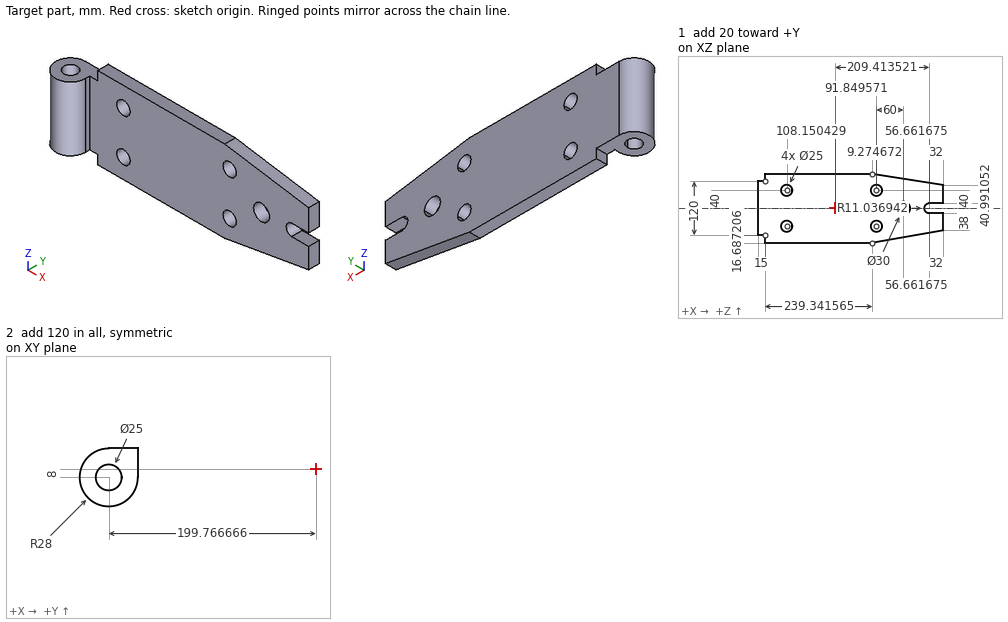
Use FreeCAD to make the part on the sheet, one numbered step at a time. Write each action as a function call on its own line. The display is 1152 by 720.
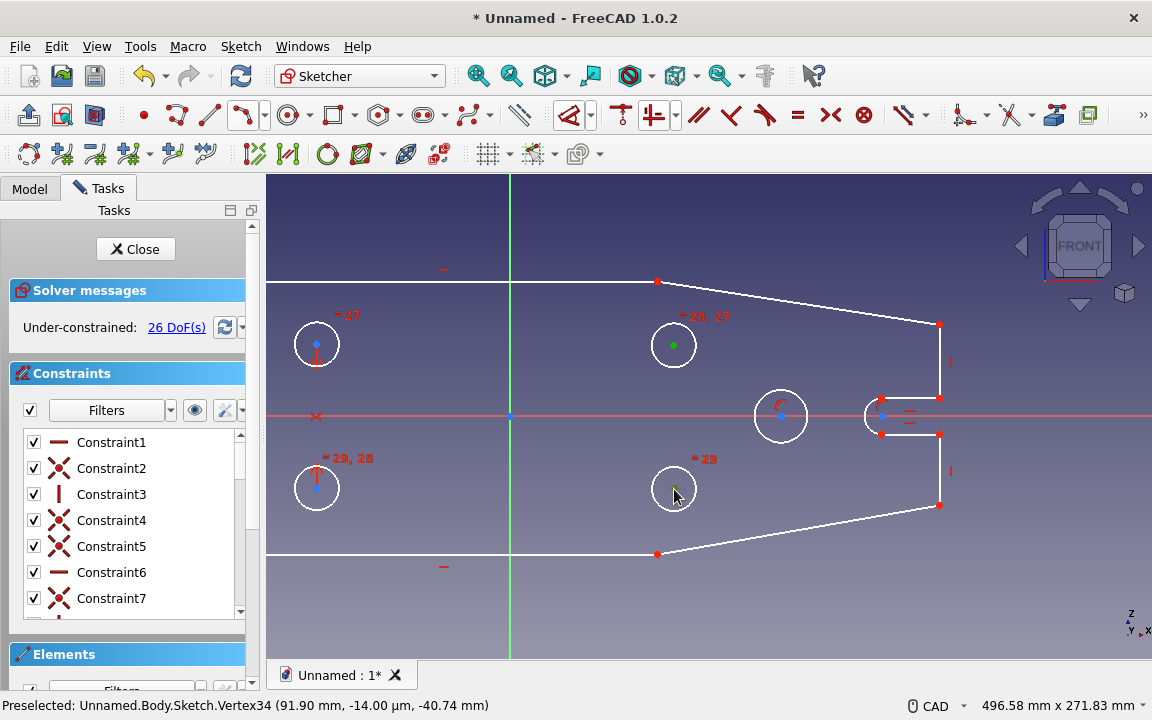
click(344, 416)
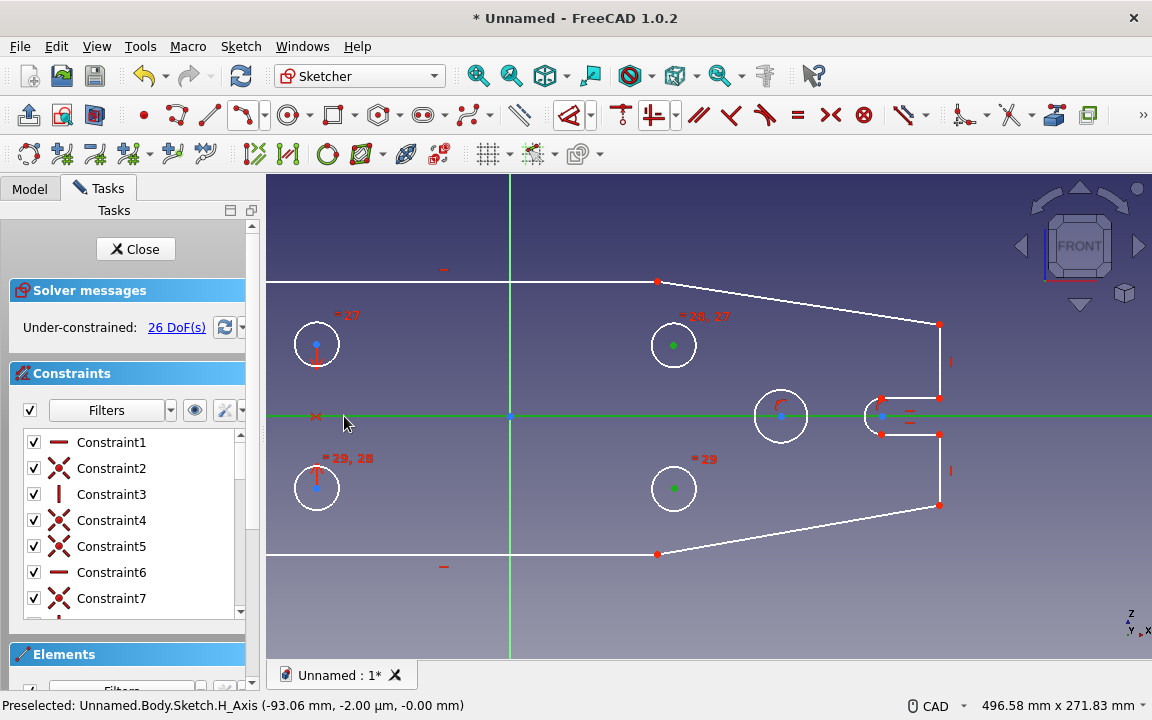
click(831, 116)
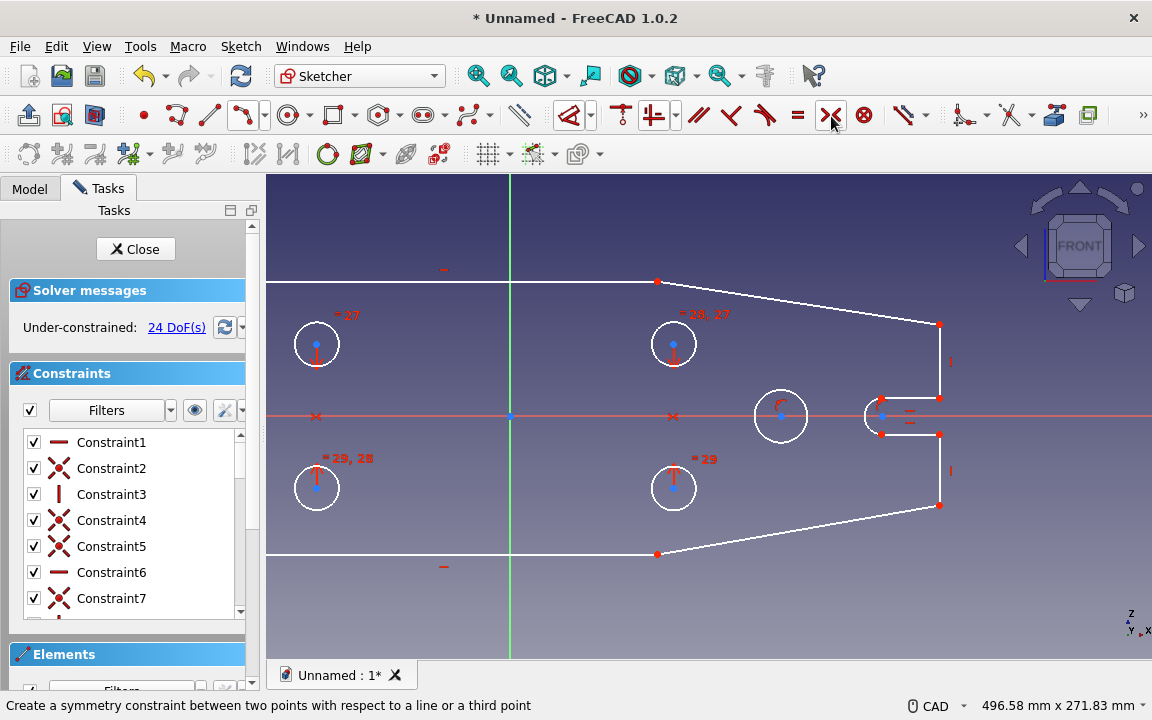
scroll(781, 417, down, 2)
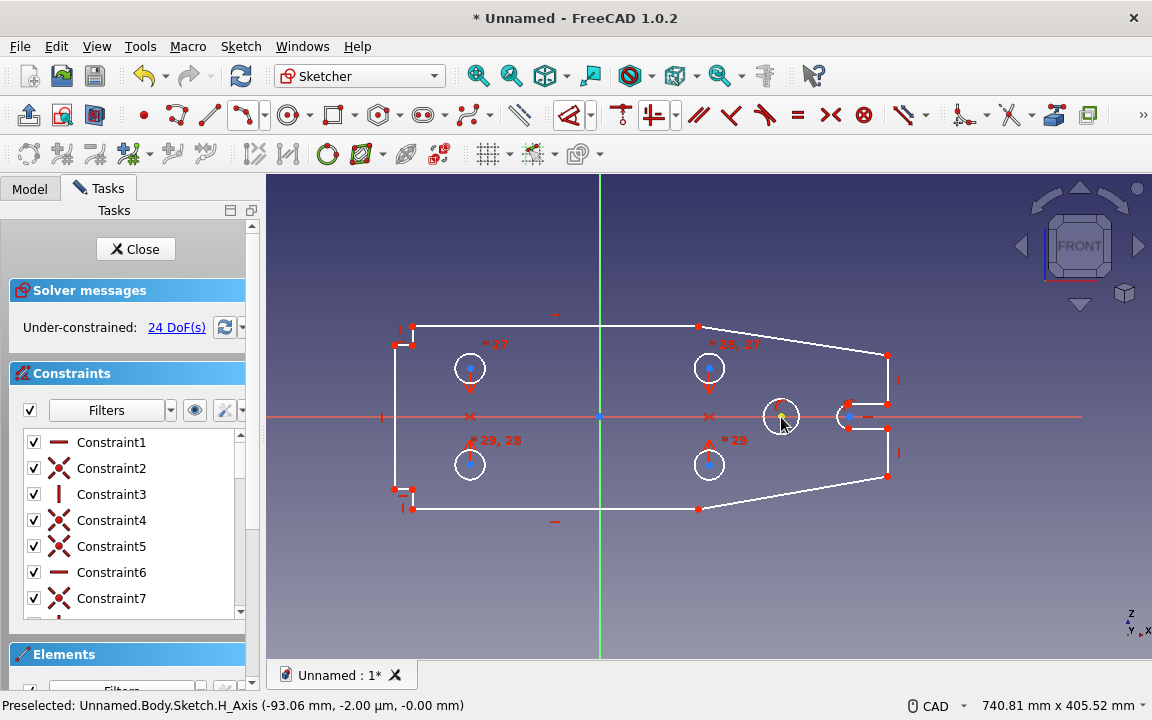
click(413, 489)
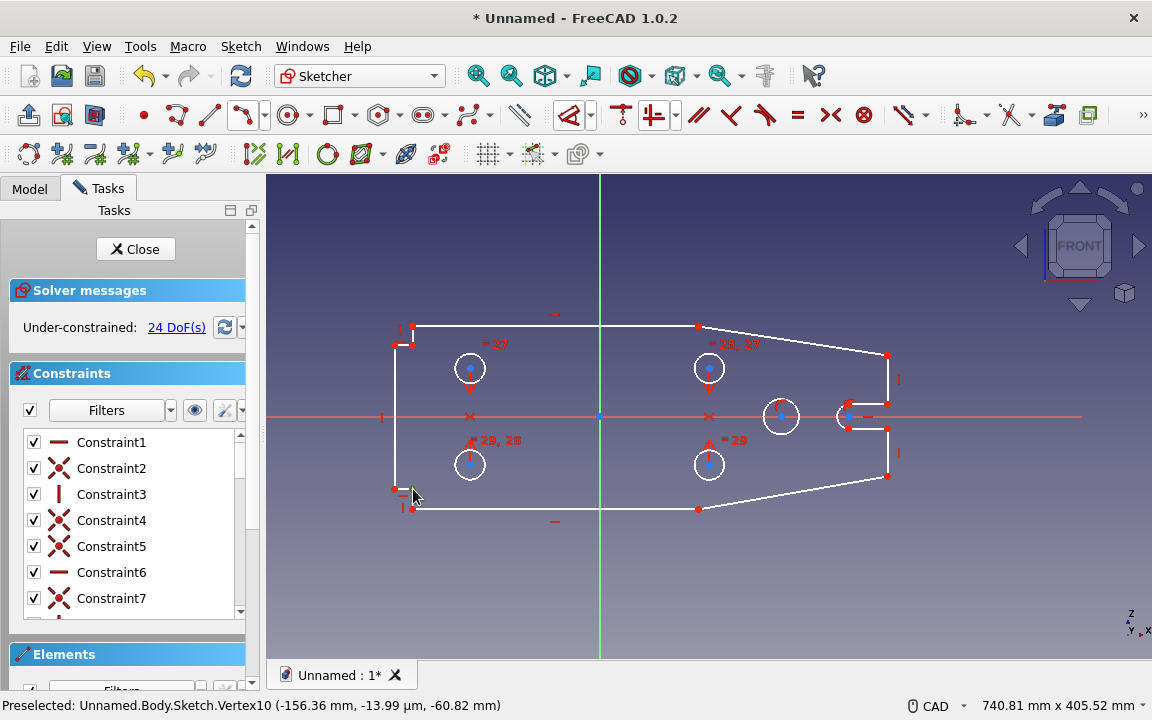
click(413, 345)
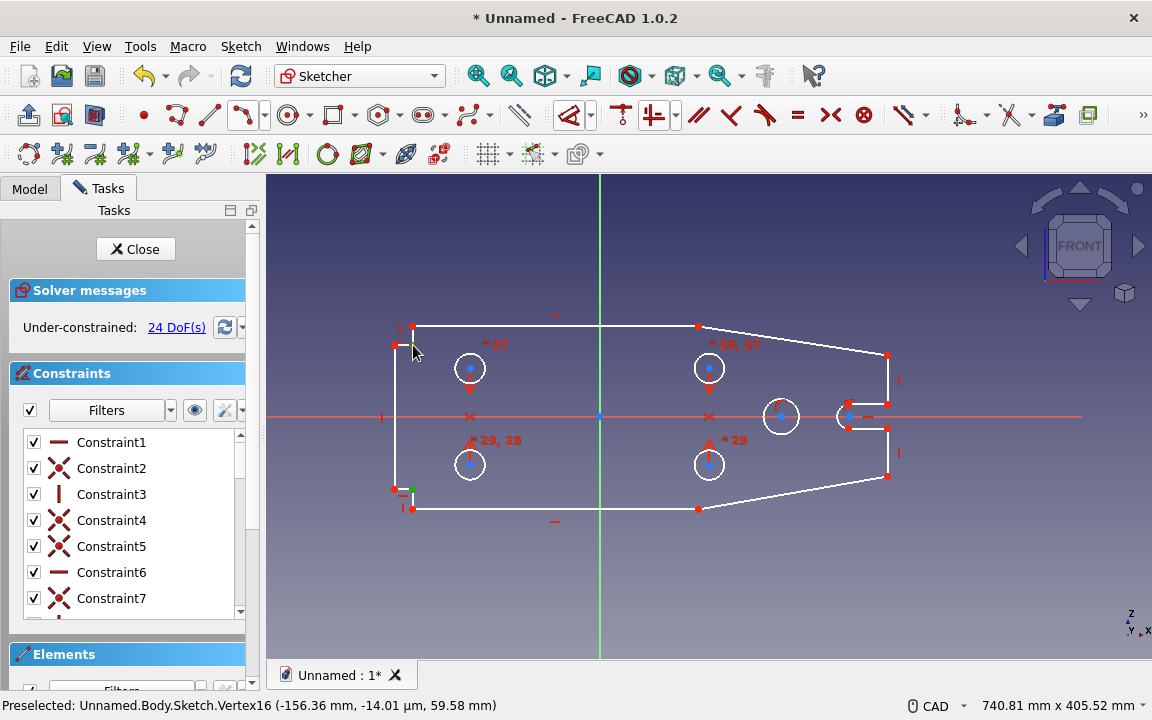
click(344, 417)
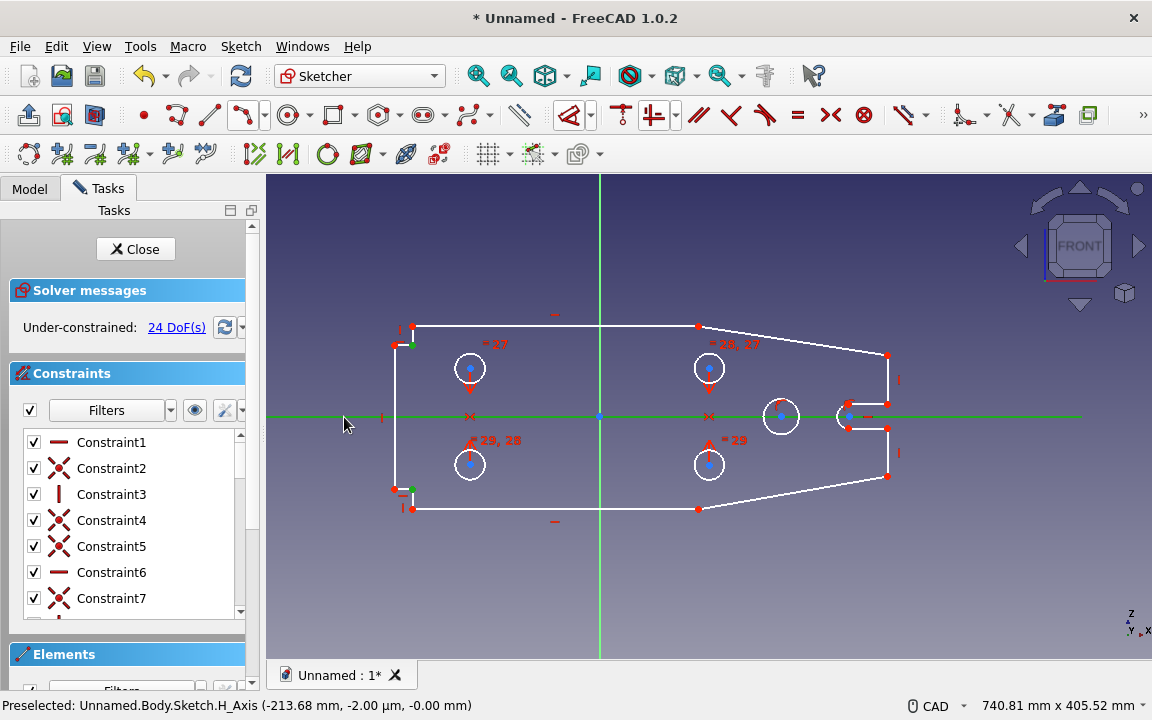
click(831, 116)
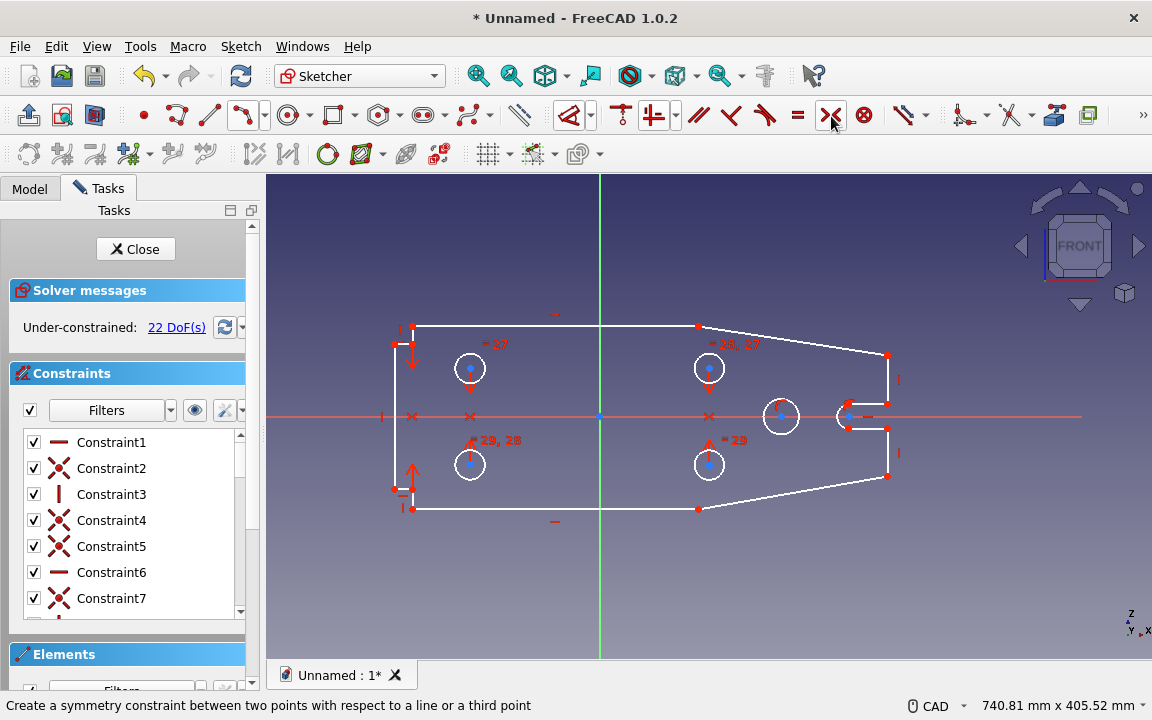
click(699, 509)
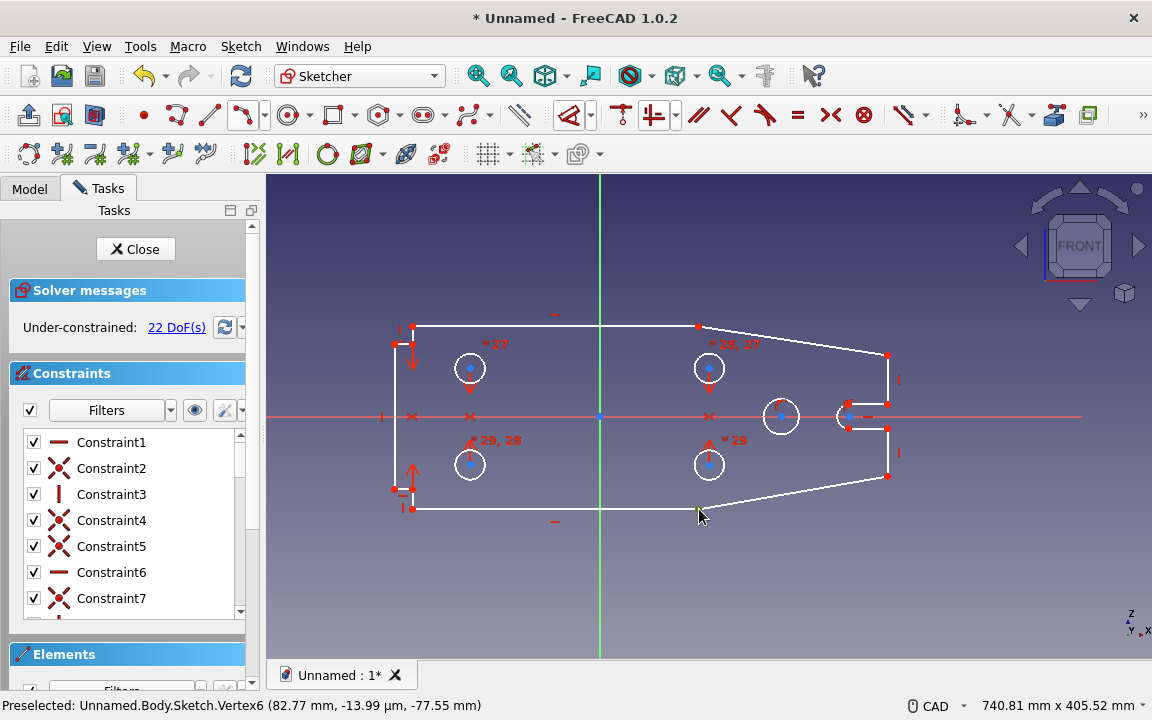
click(699, 326)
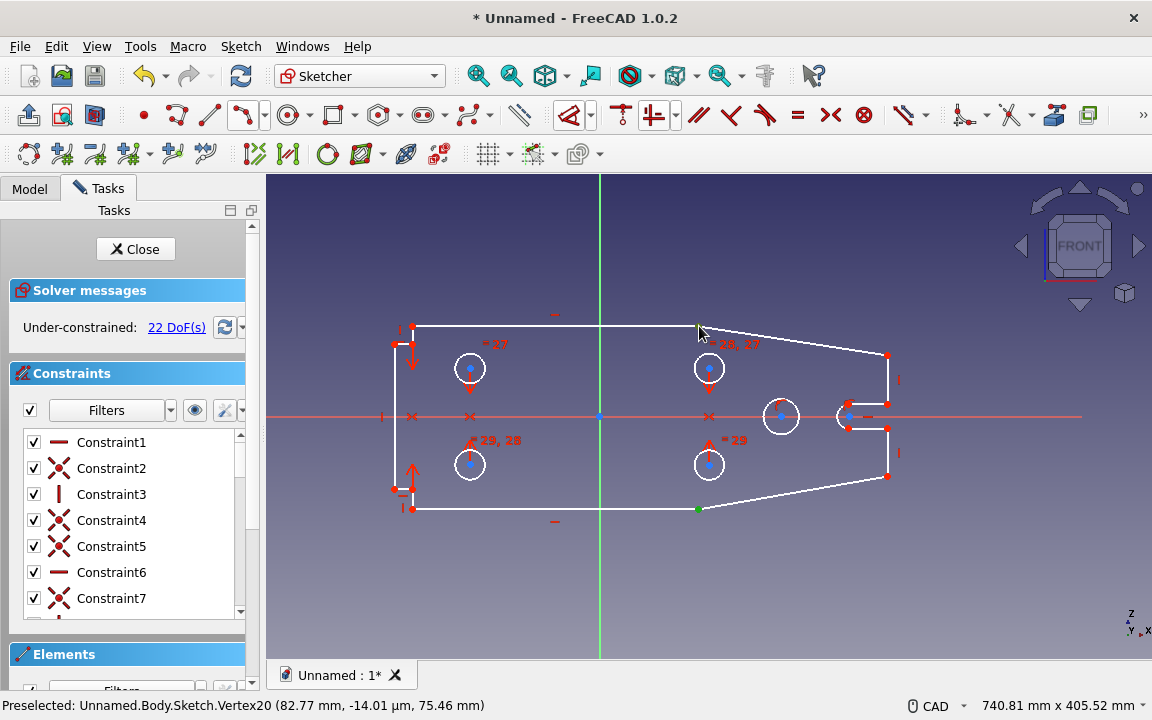
click(344, 417)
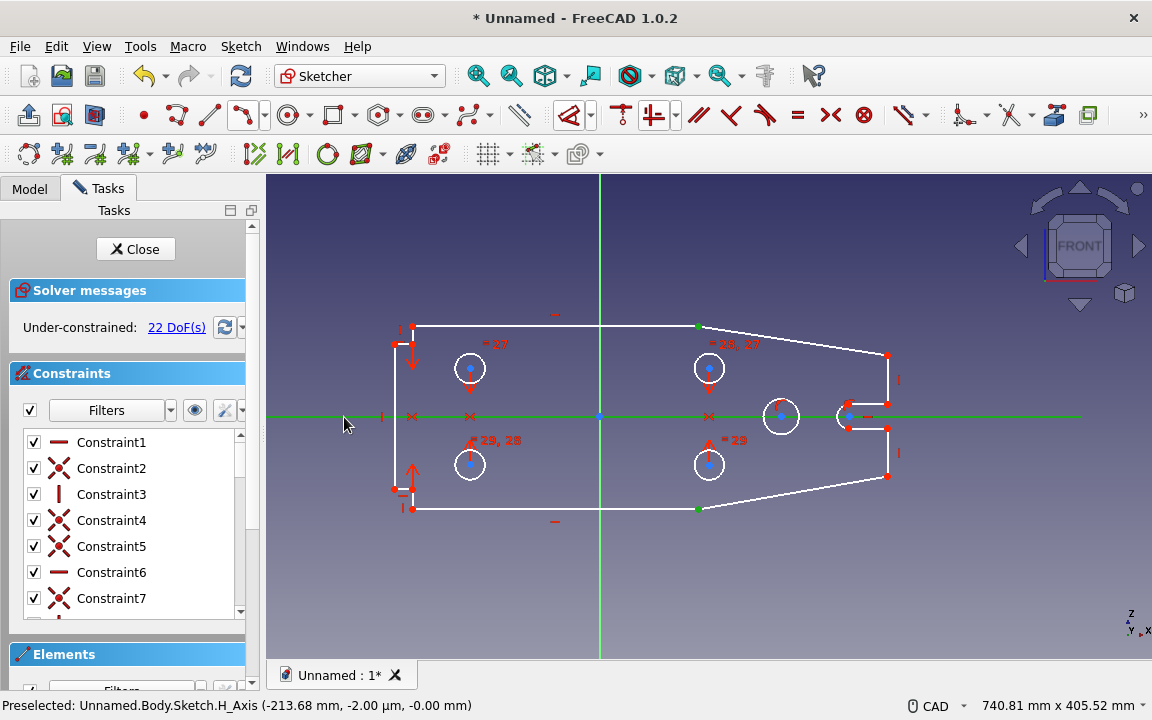
key(s)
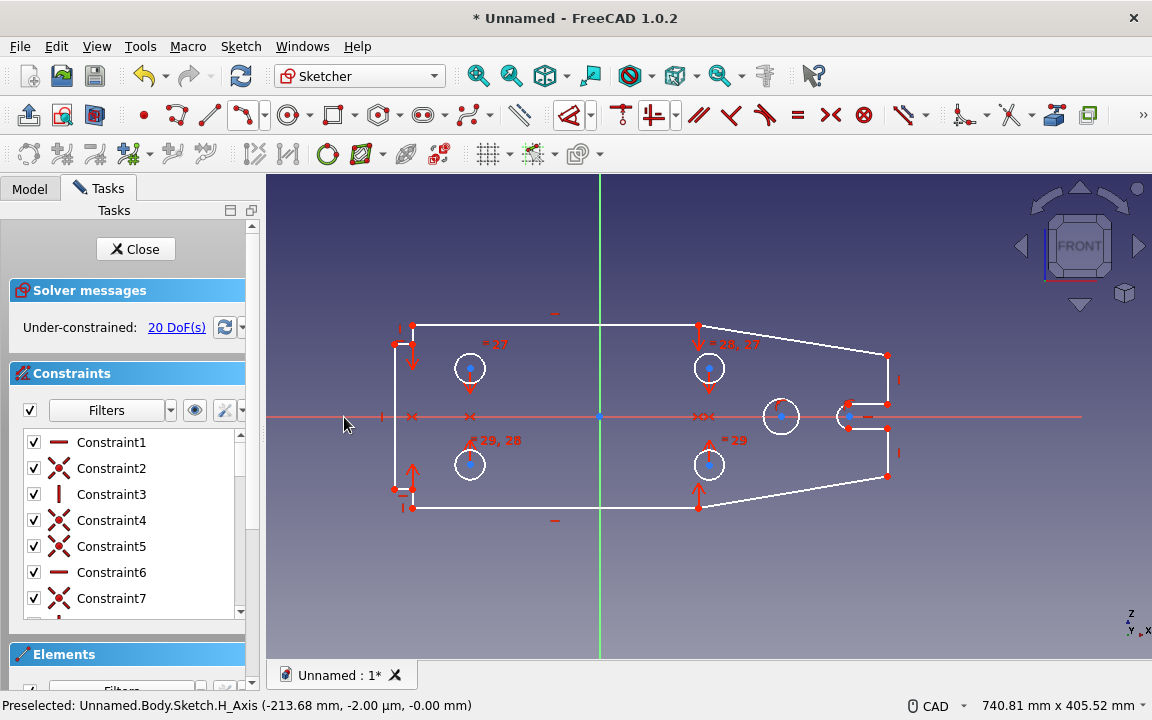
click(568, 116)